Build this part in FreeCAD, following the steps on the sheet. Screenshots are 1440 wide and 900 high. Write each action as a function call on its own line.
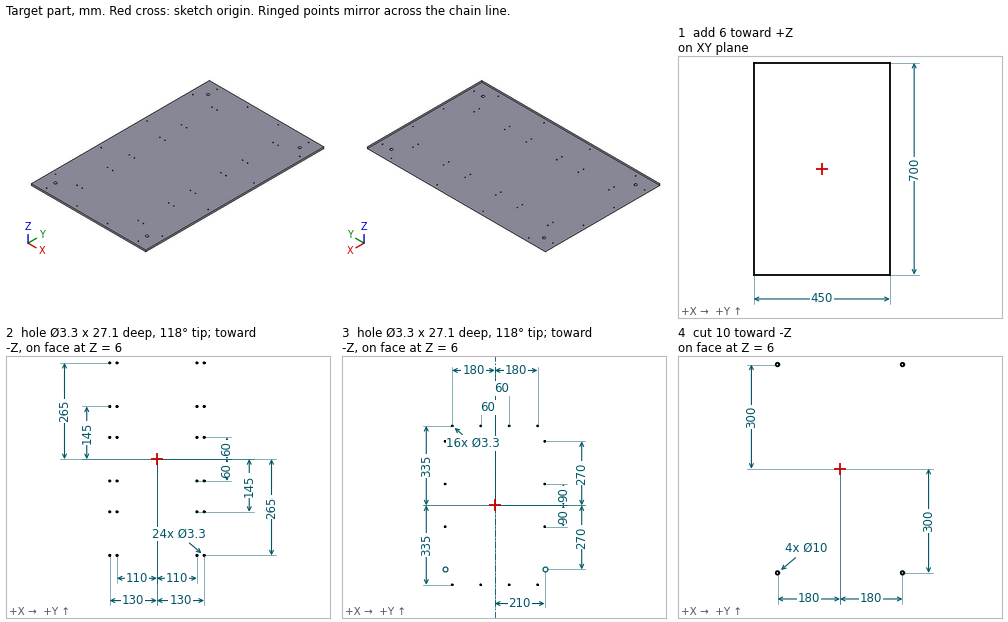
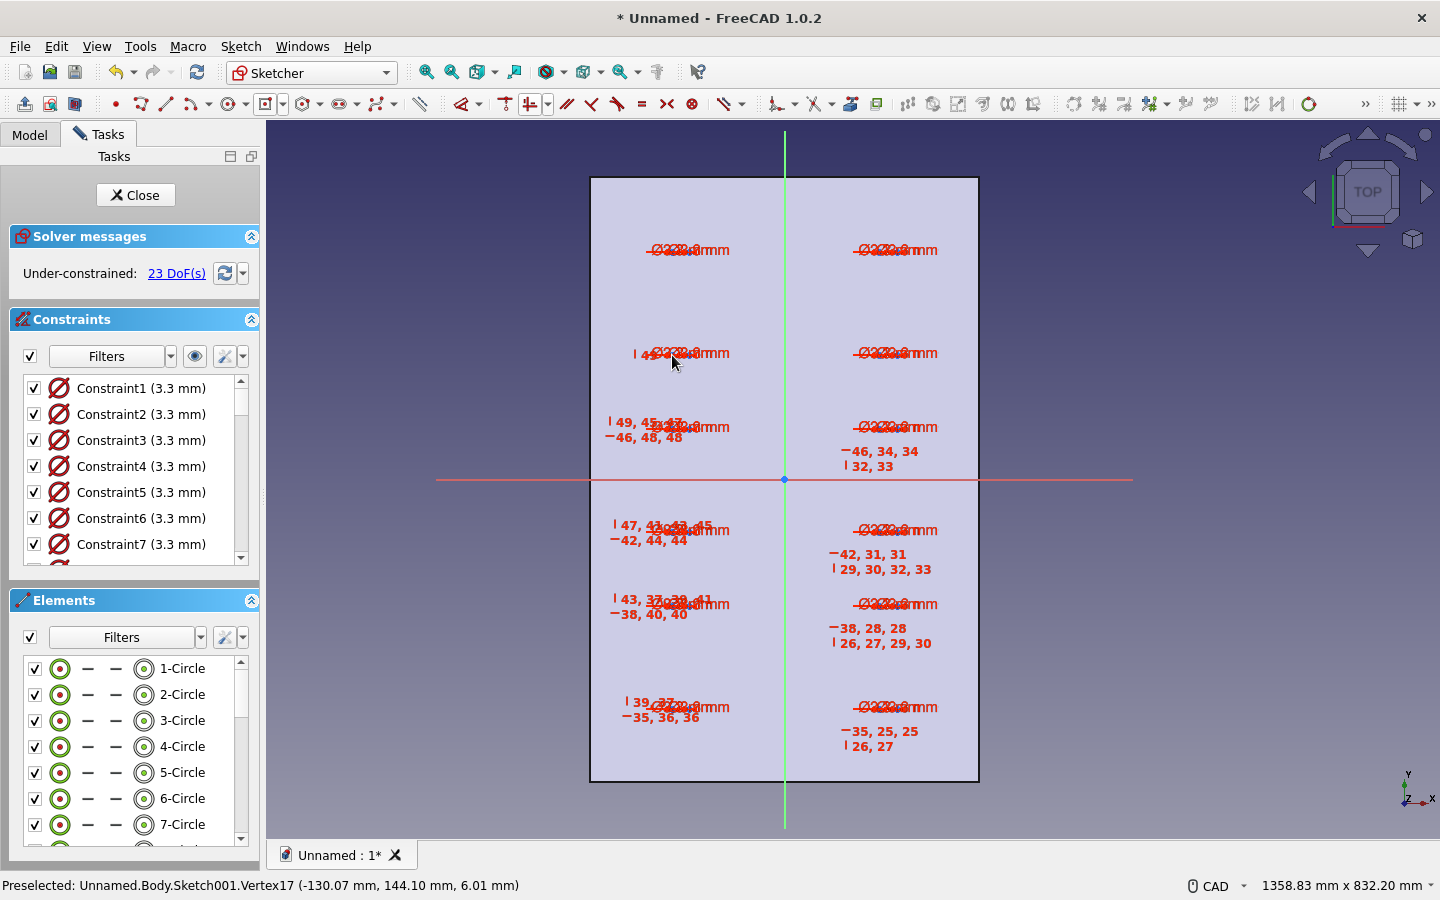
click(689, 429)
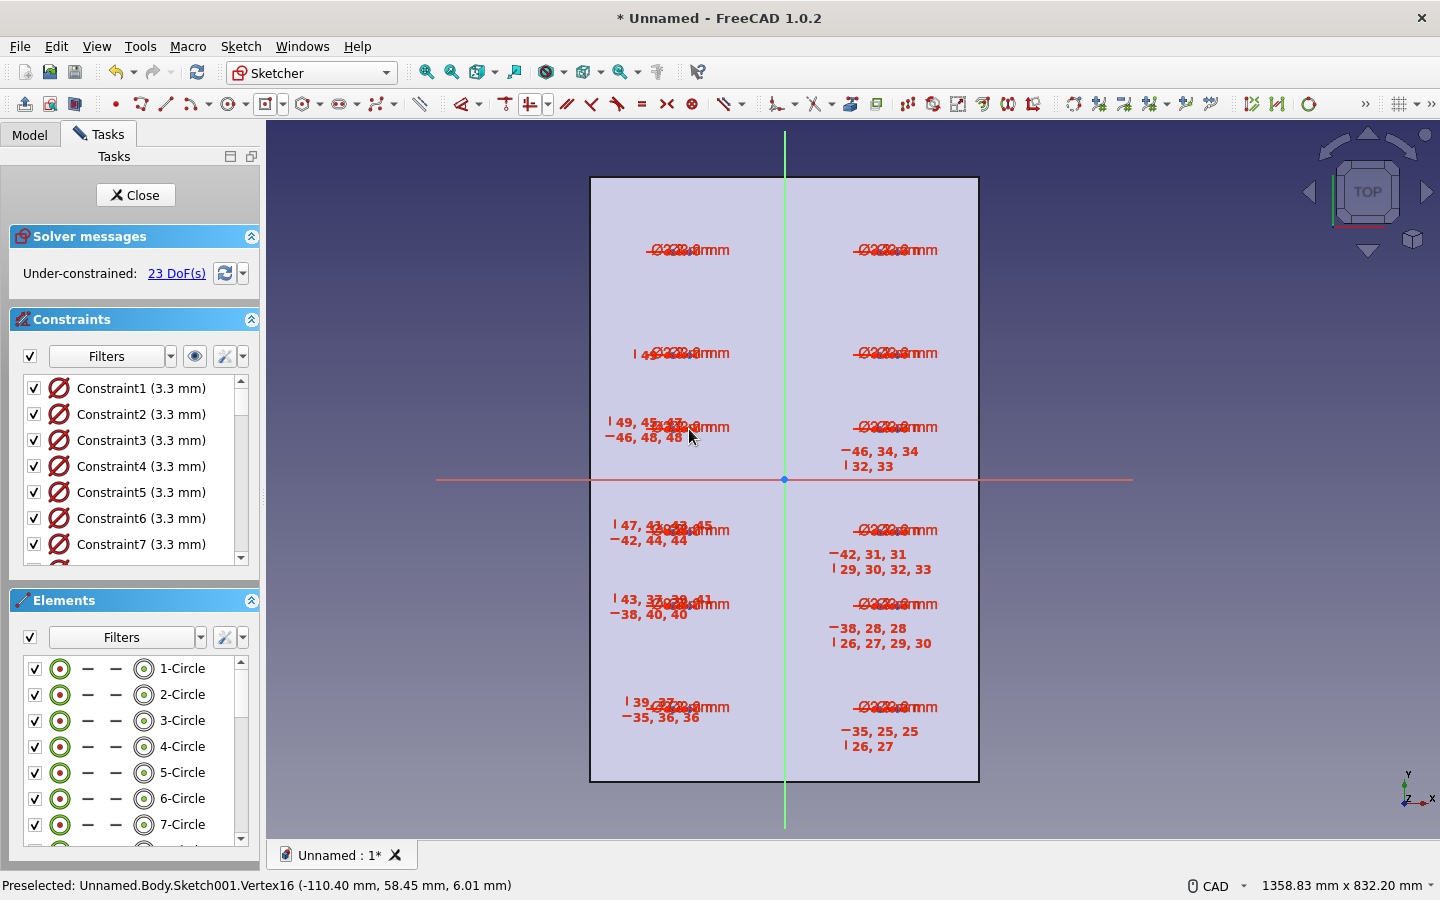
click(689, 355)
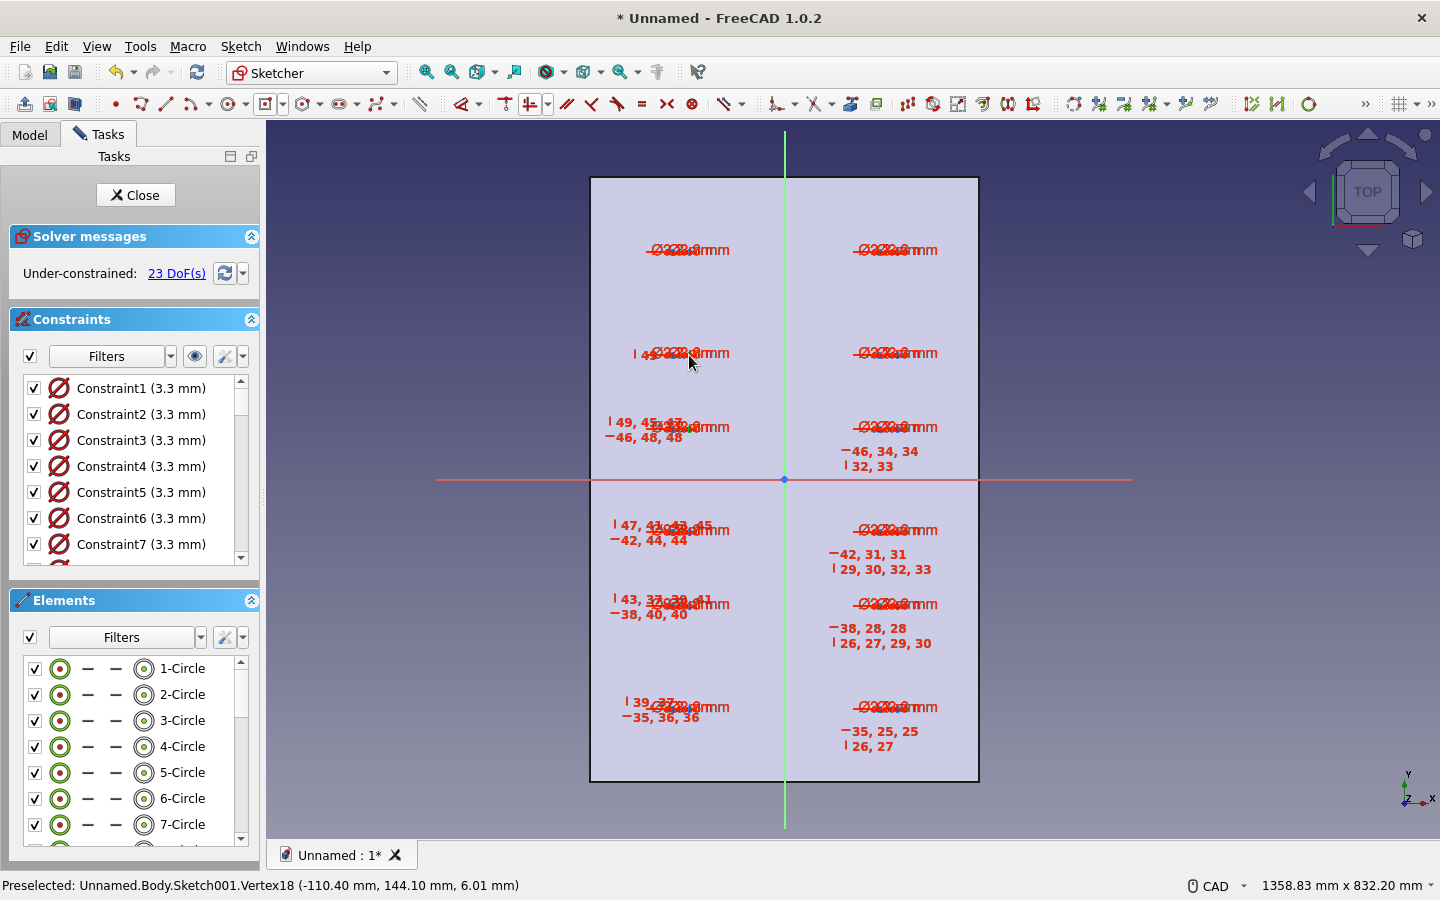
click(548, 104)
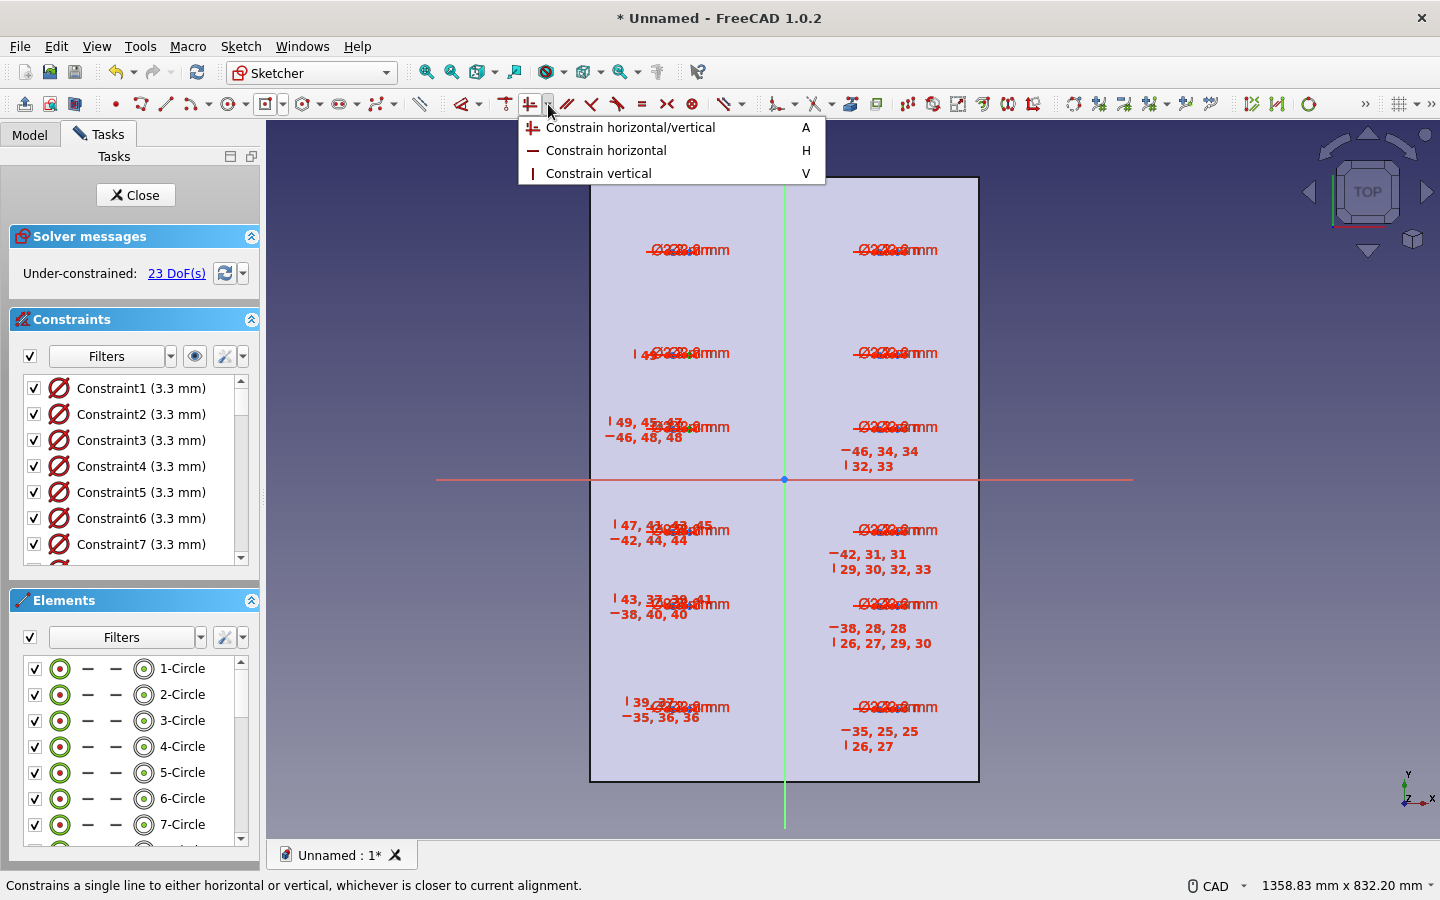
click(672, 174)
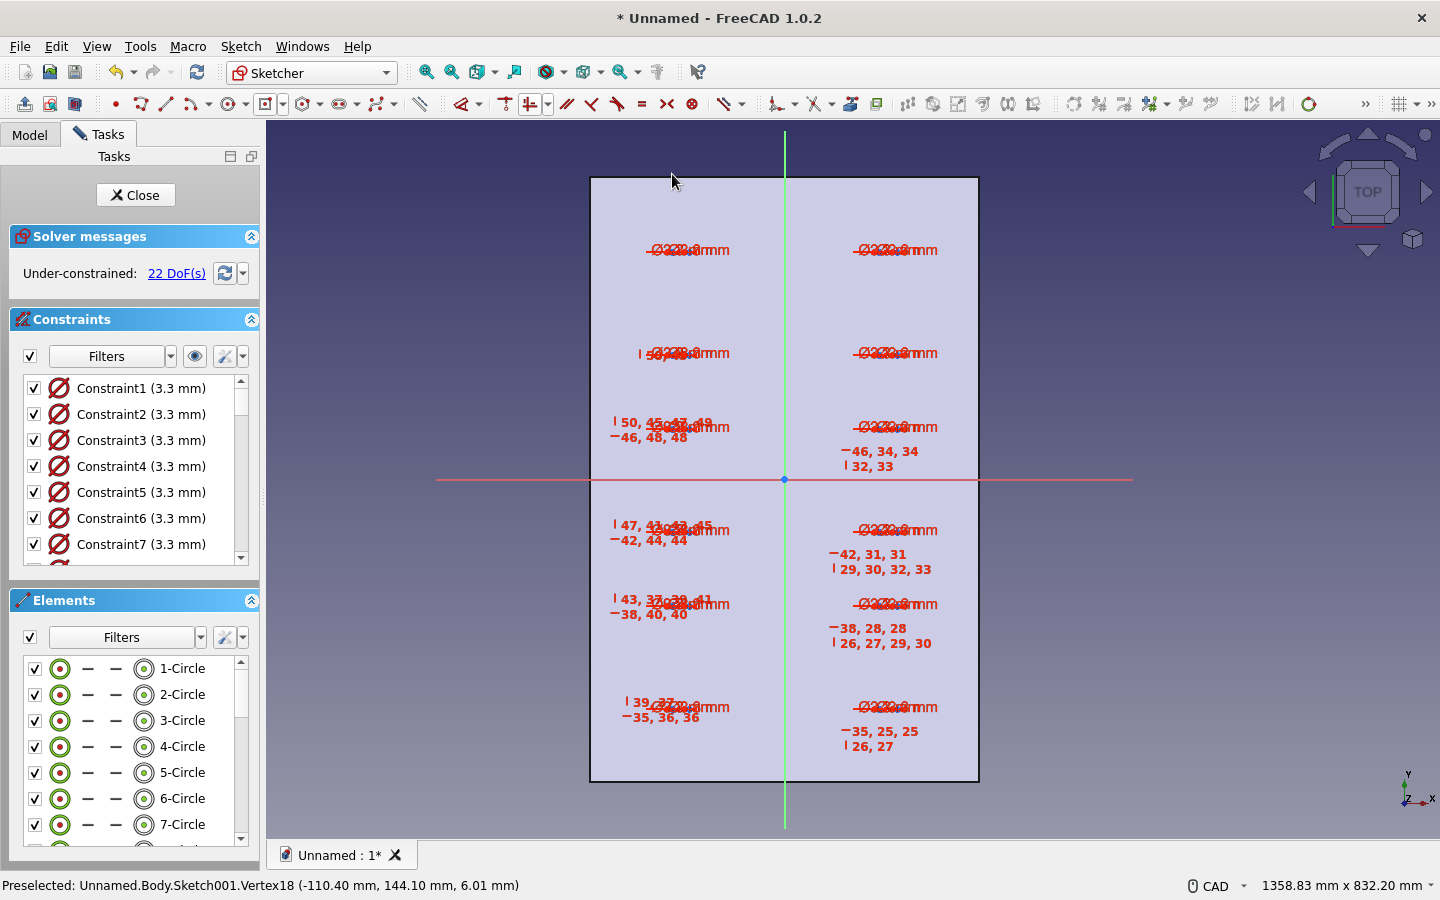
scroll(672, 355, up, 4)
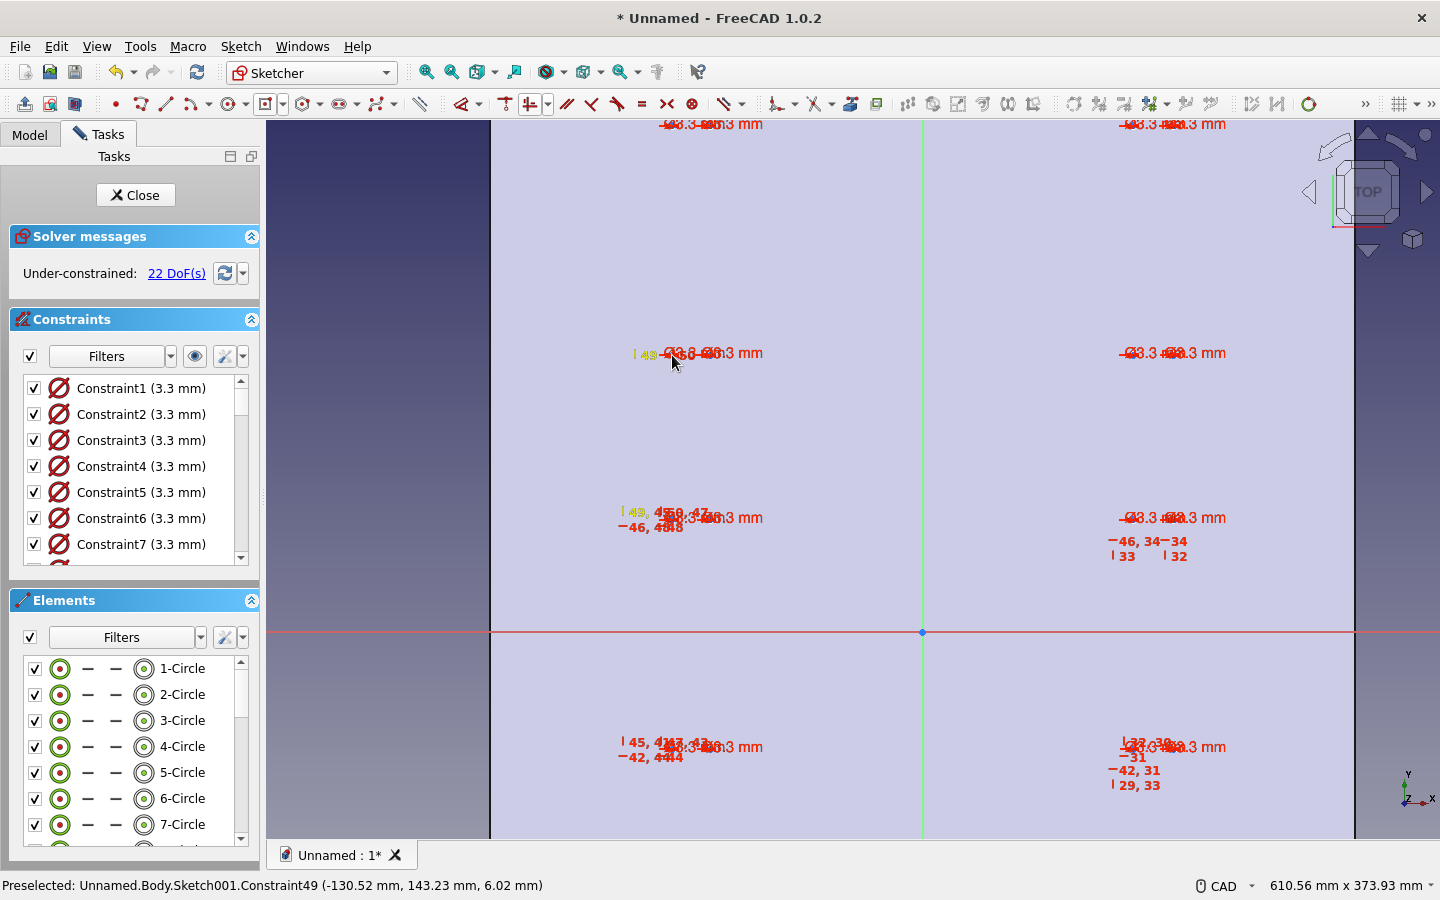
scroll(672, 355, up, 4)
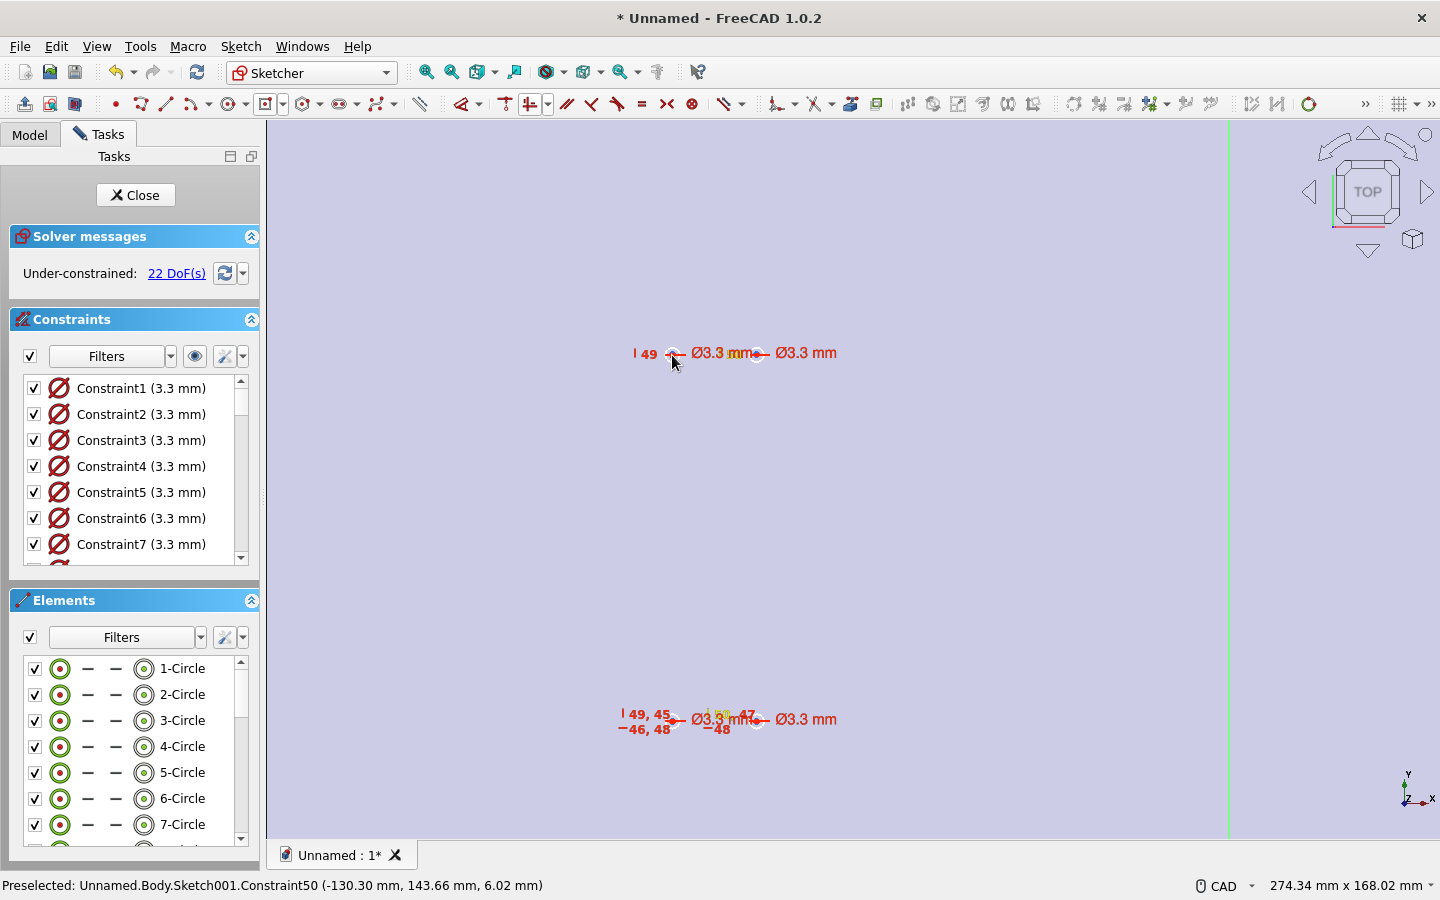
click(673, 355)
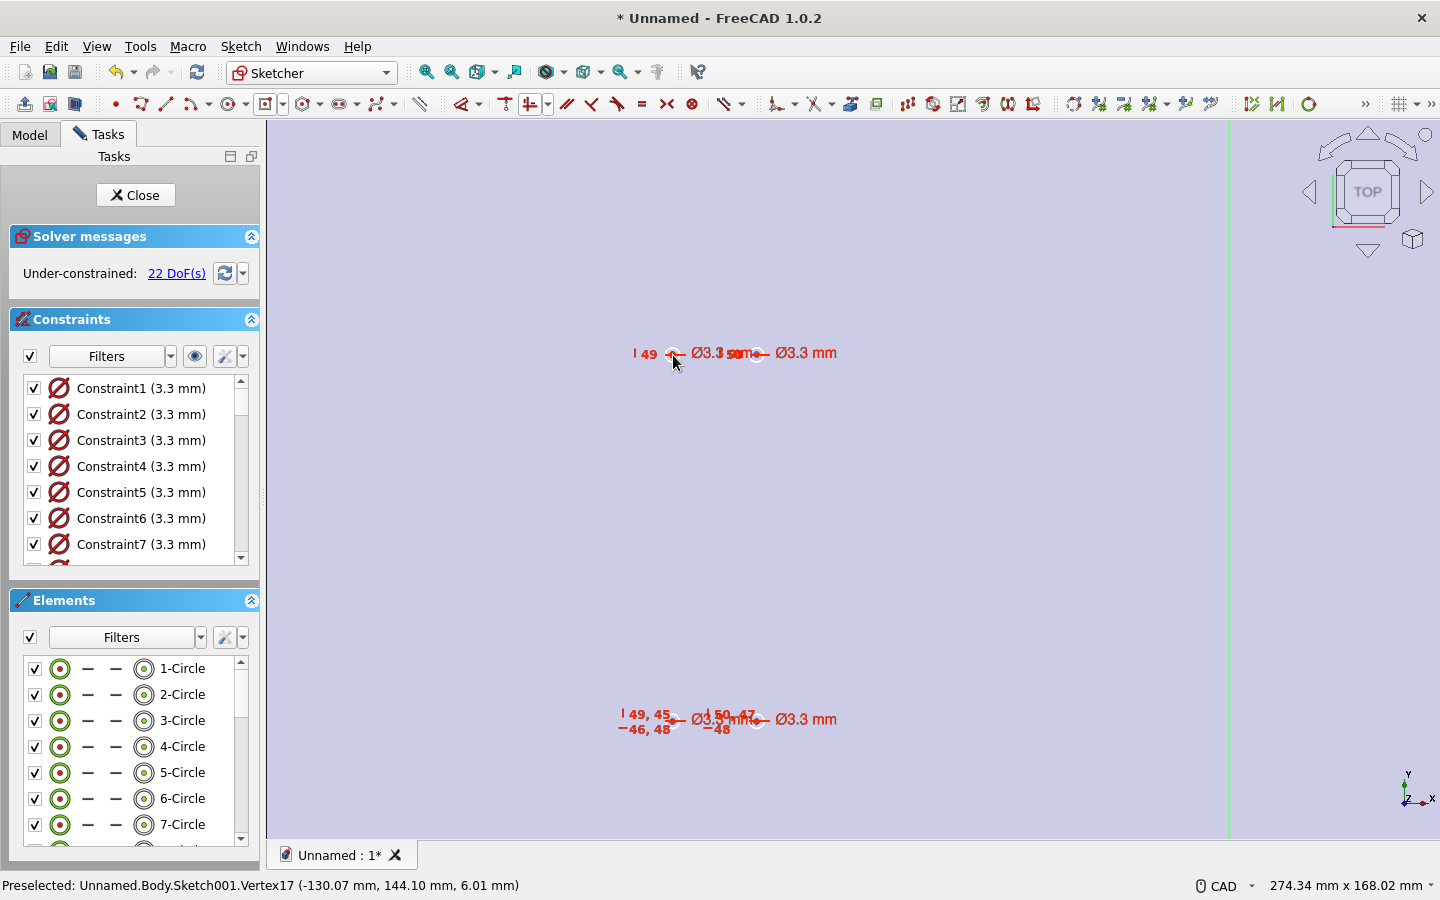
scroll(672, 355, down, 8)